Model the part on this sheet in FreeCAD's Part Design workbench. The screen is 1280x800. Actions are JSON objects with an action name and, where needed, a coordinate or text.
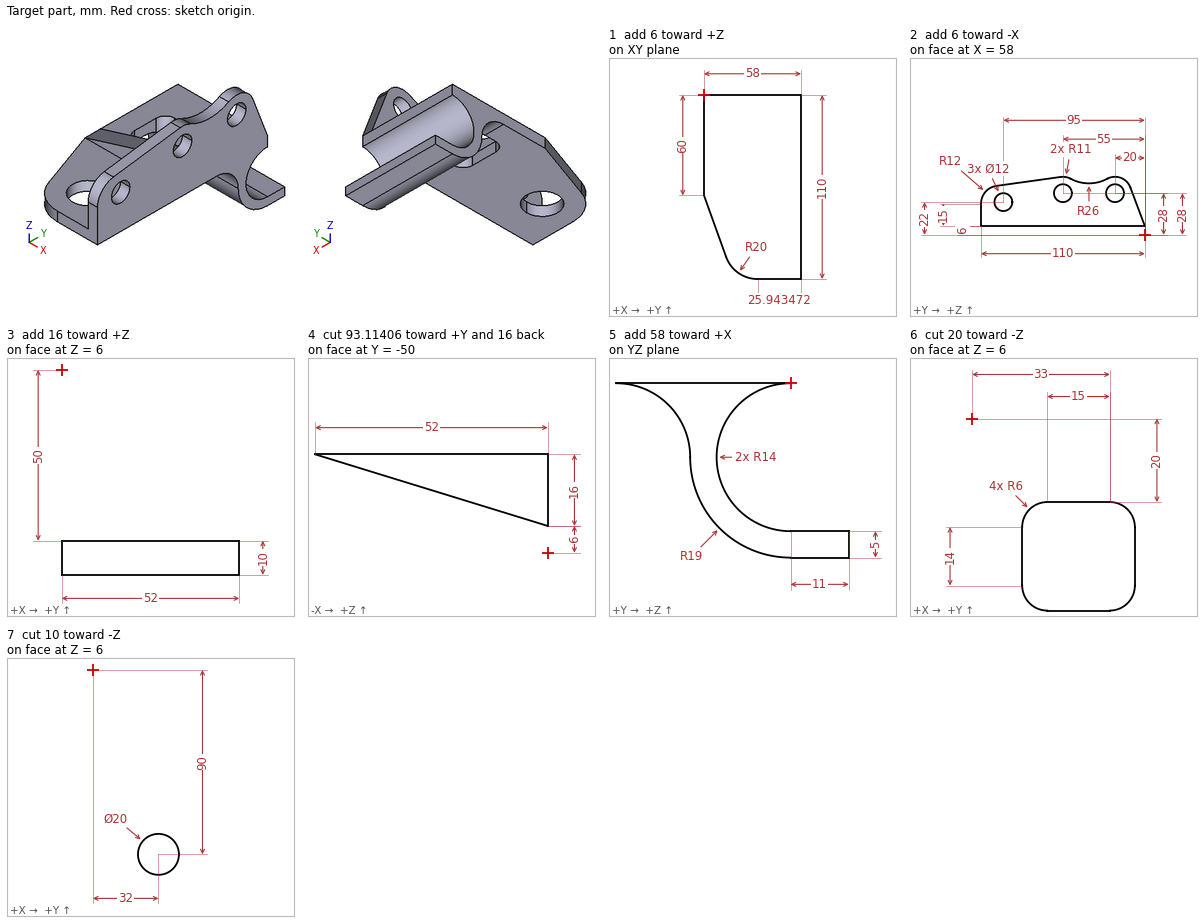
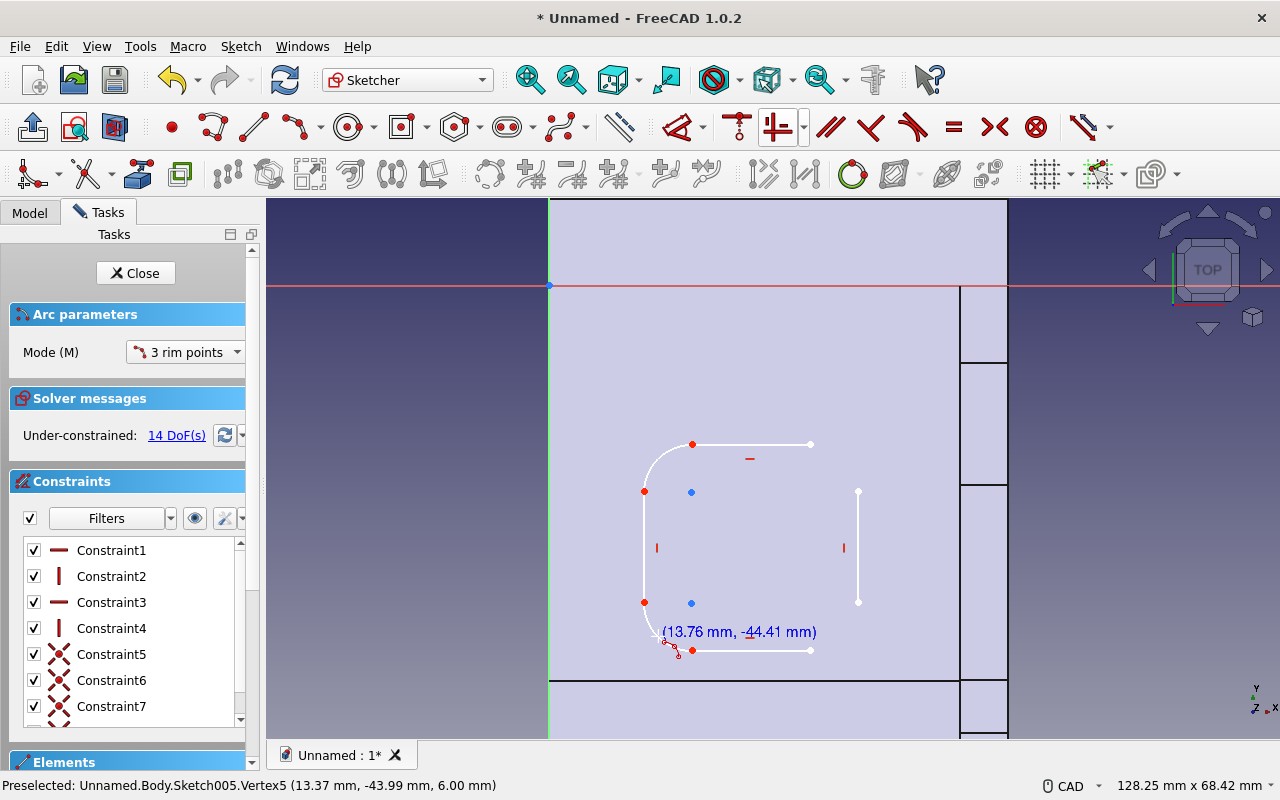
{"action": "left_click", "coordinate": [810, 651]}
{"action": "left_click", "coordinate": [858, 603]}
{"action": "left_click", "coordinate": [844, 636]}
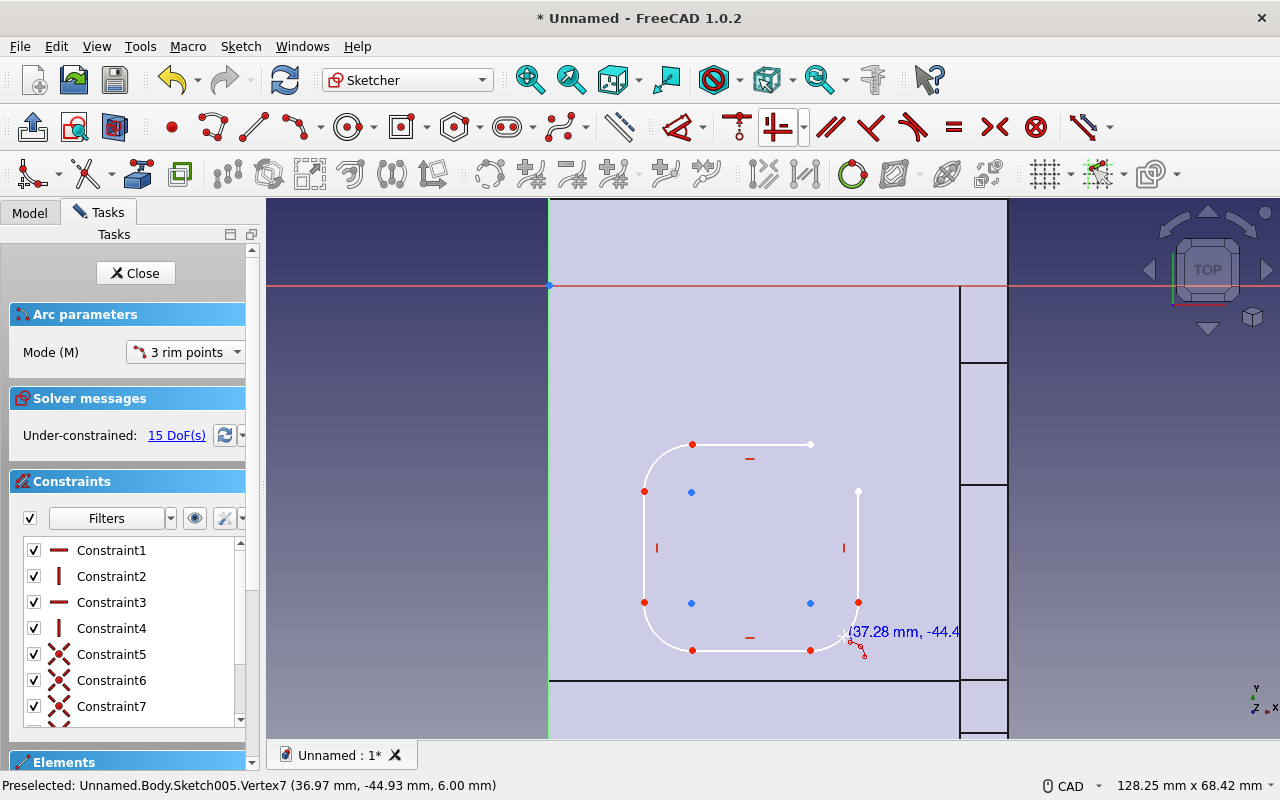
{"action": "left_click", "coordinate": [858, 492]}
{"action": "left_click", "coordinate": [810, 445]}
{"action": "left_click", "coordinate": [844, 458]}
{"action": "key", "text": "Escape"}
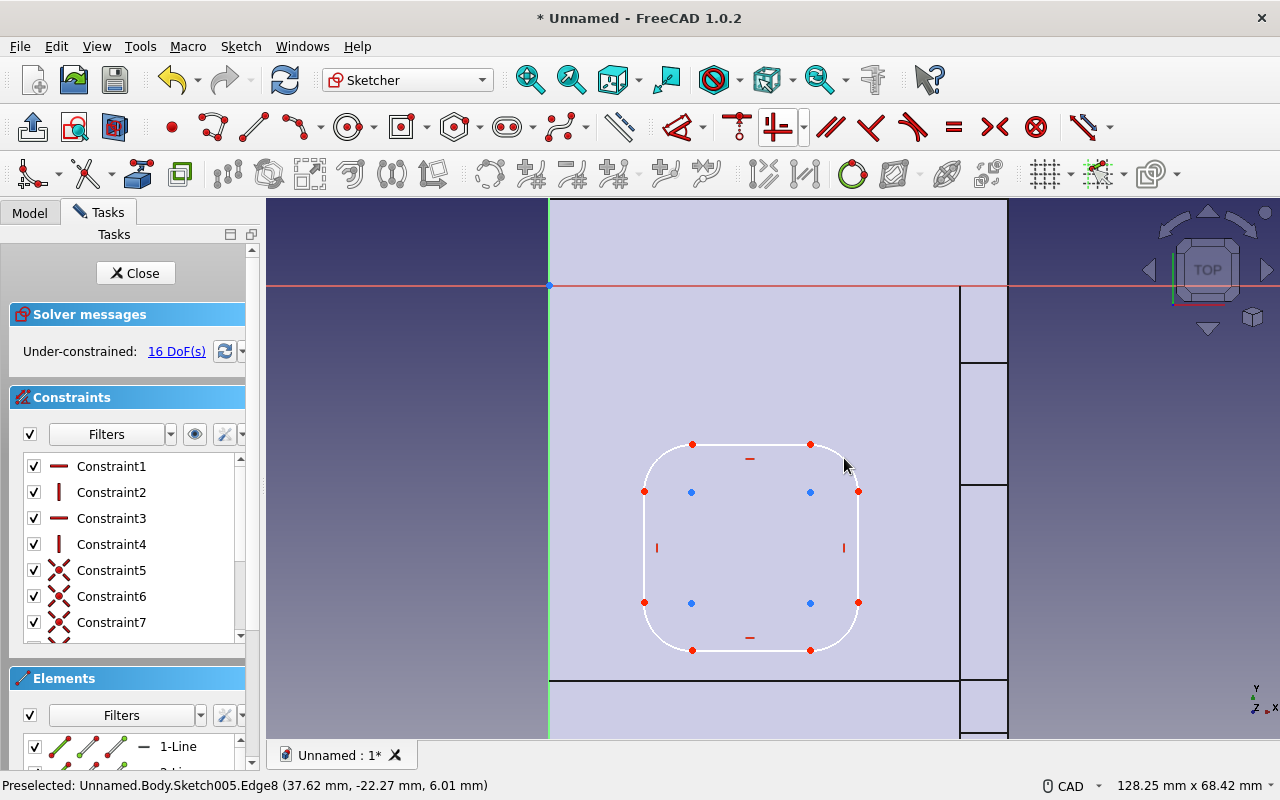
{"action": "left_click", "coordinate": [775, 445]}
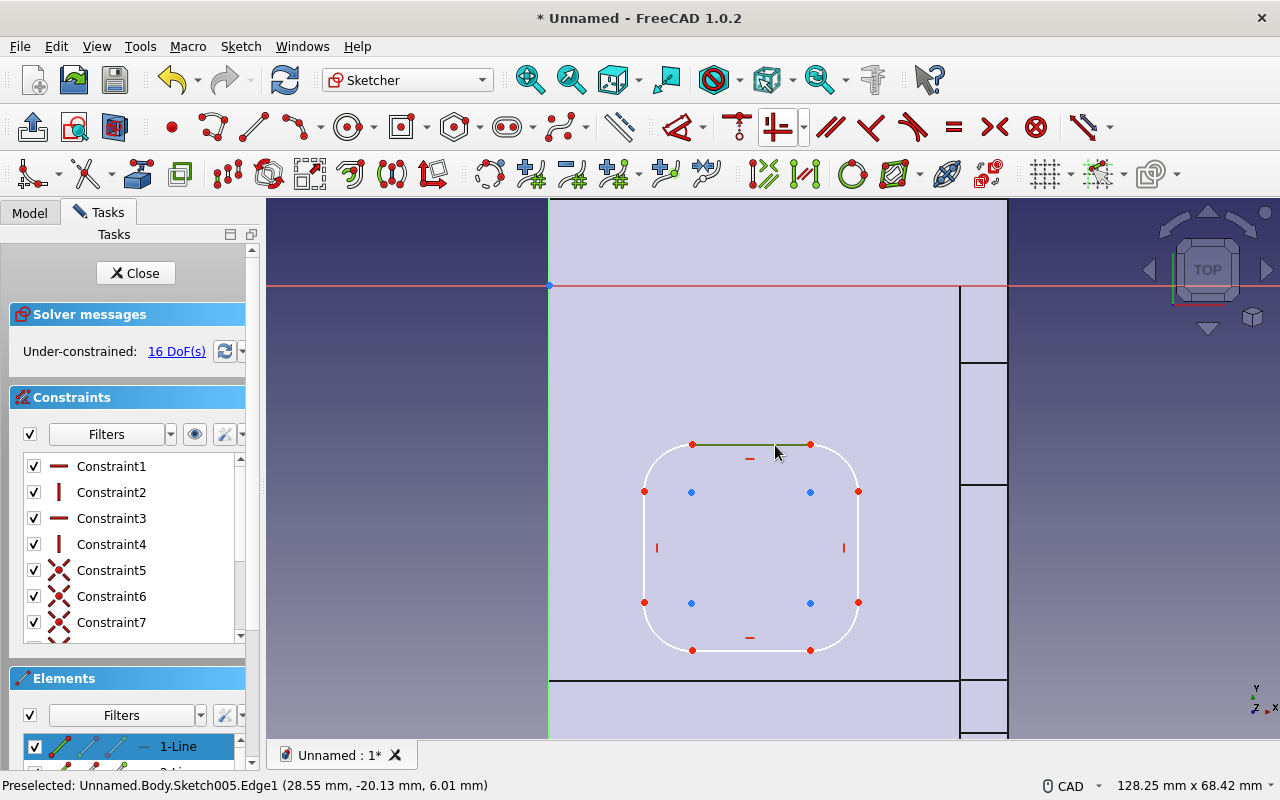
{"action": "left_click", "coordinate": [670, 450]}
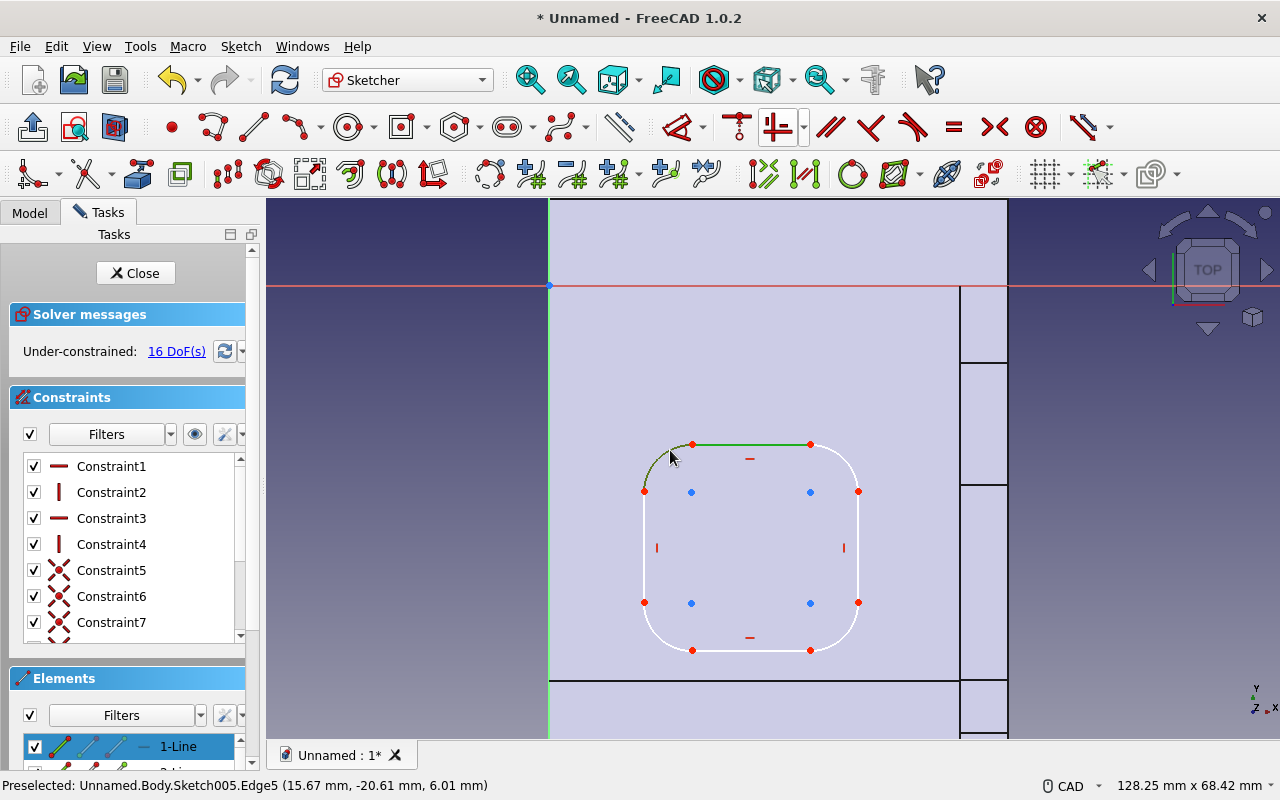
{"action": "left_click", "coordinate": [913, 128]}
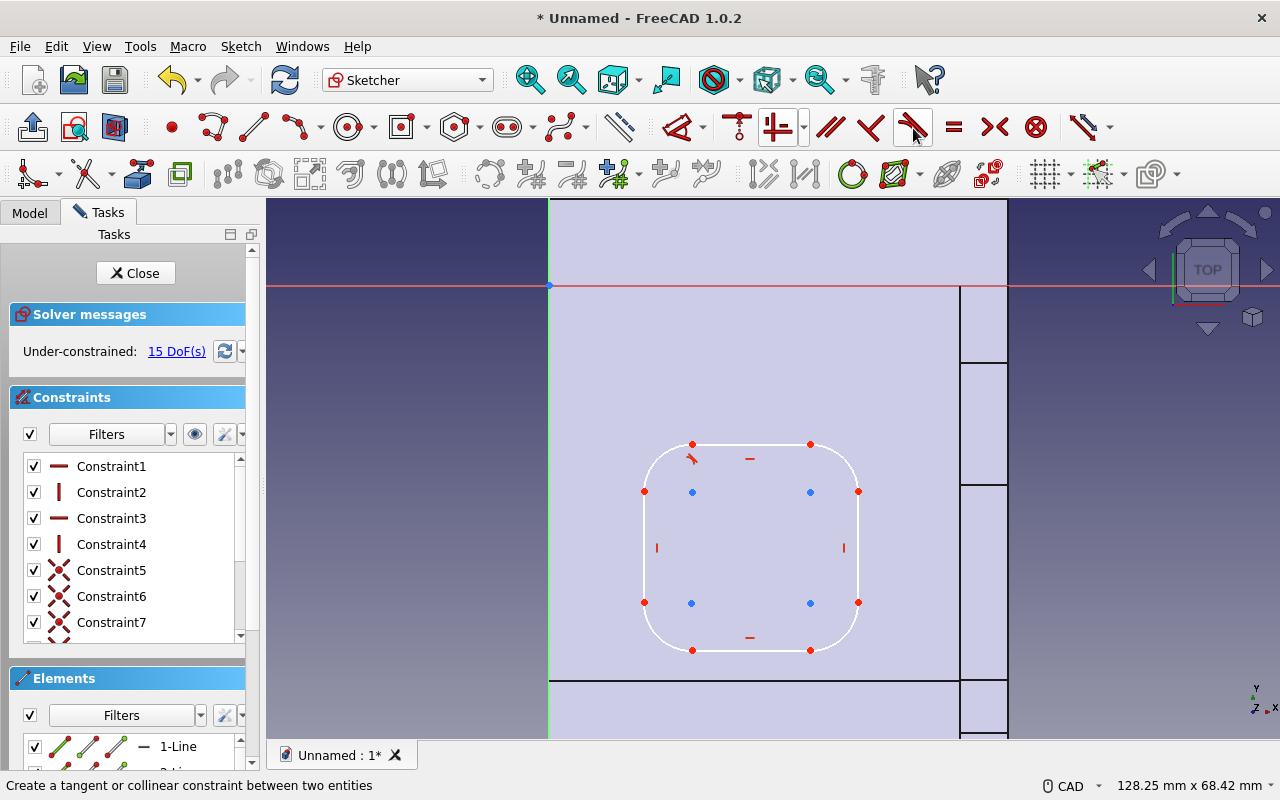
{"action": "left_click", "coordinate": [775, 445]}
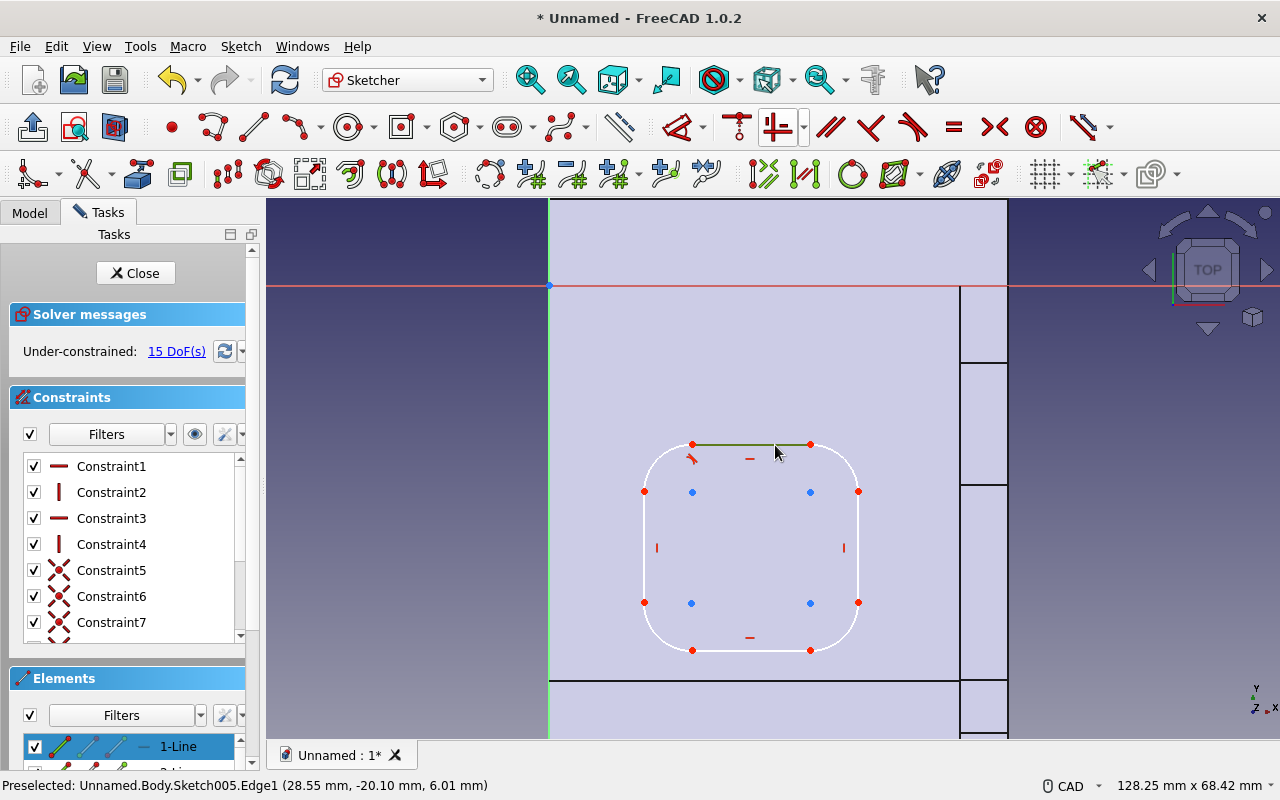
{"action": "left_click", "coordinate": [853, 471]}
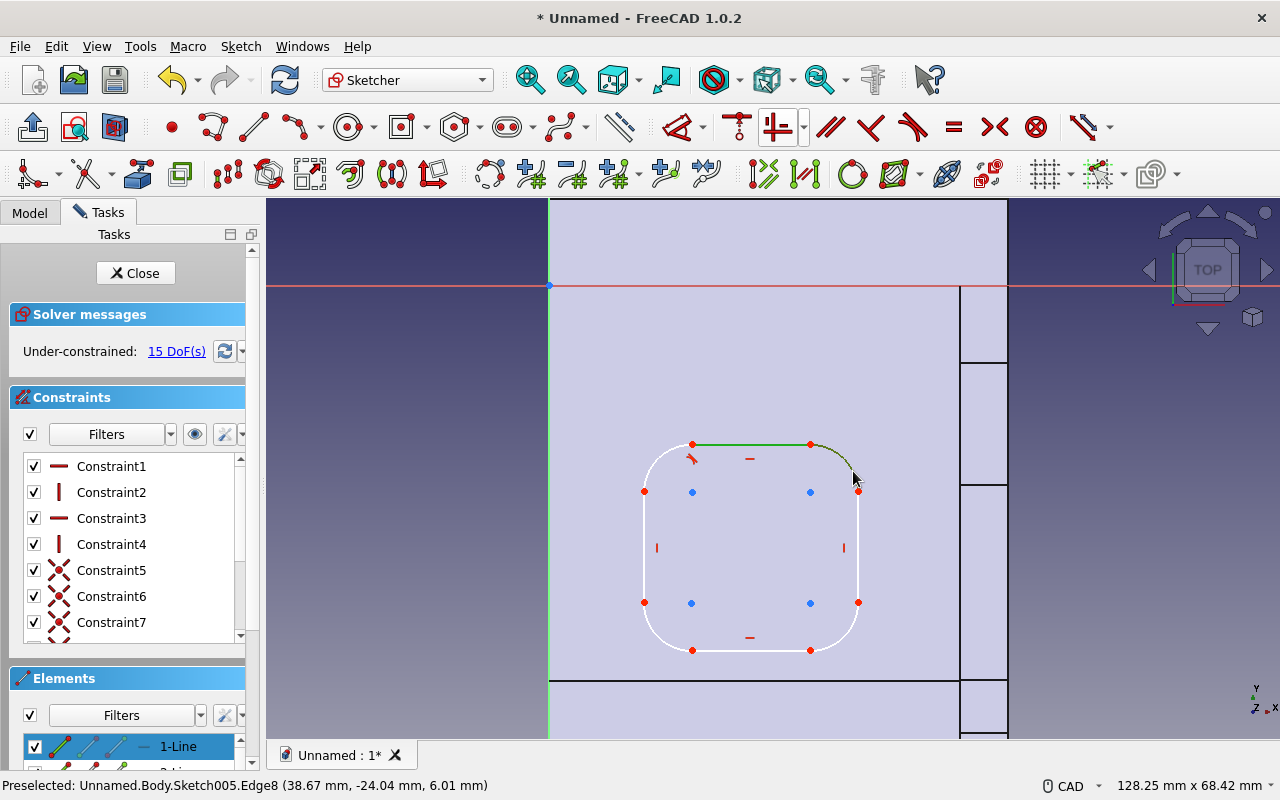
{"action": "left_click", "coordinate": [913, 128]}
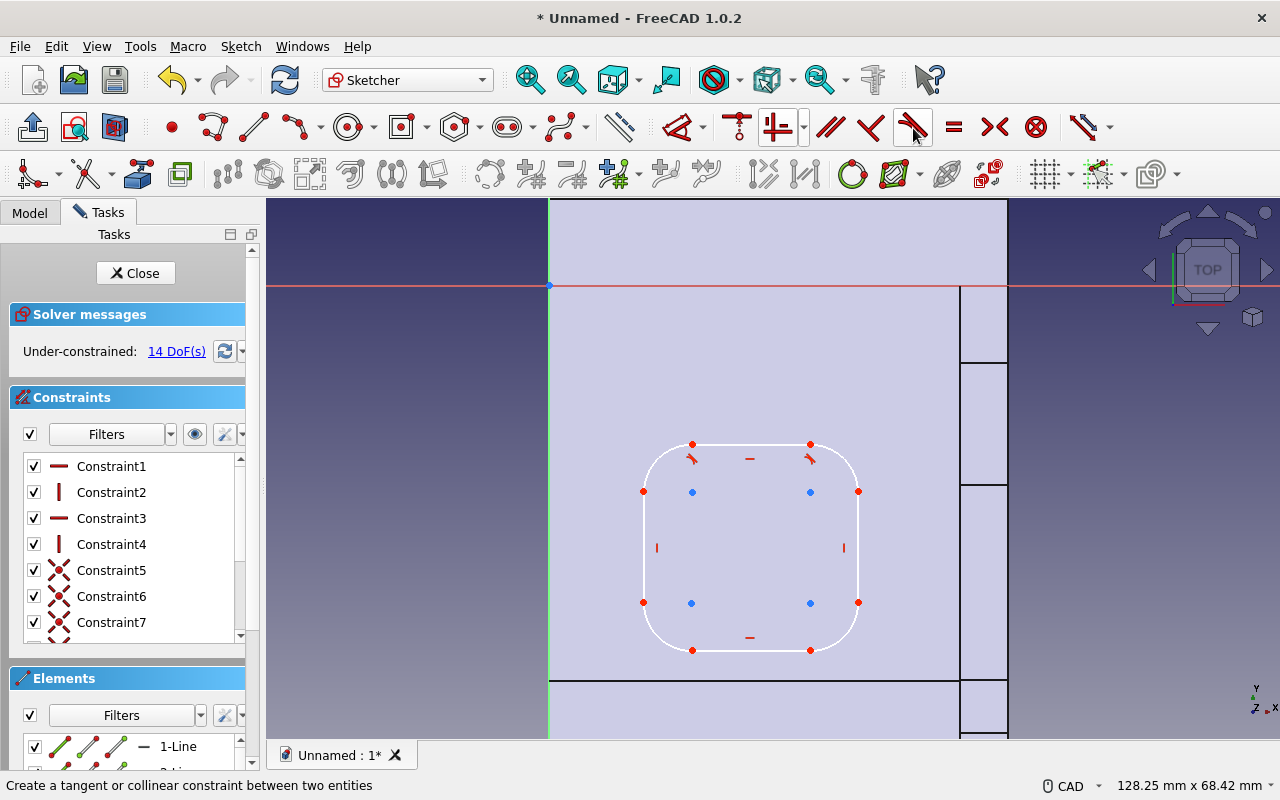
{"action": "left_click", "coordinate": [644, 525]}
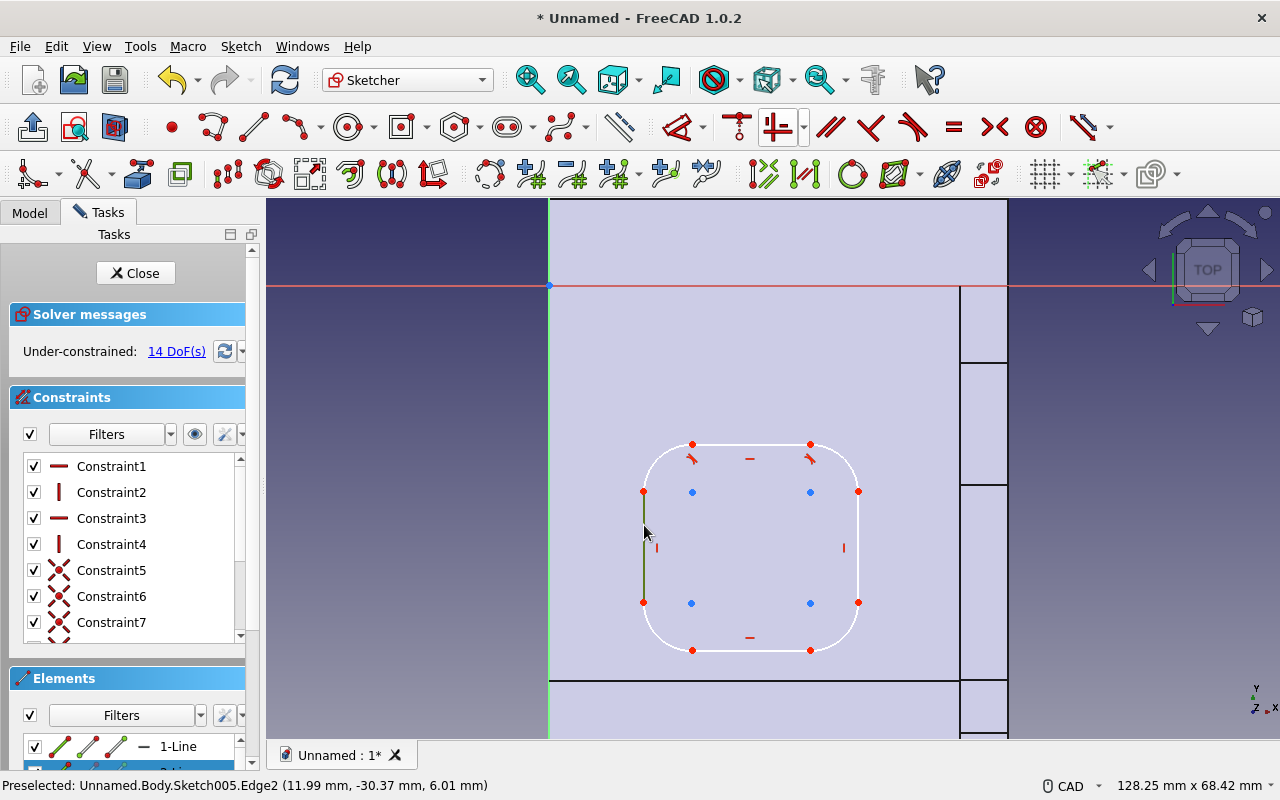
{"action": "left_click", "coordinate": [670, 450]}